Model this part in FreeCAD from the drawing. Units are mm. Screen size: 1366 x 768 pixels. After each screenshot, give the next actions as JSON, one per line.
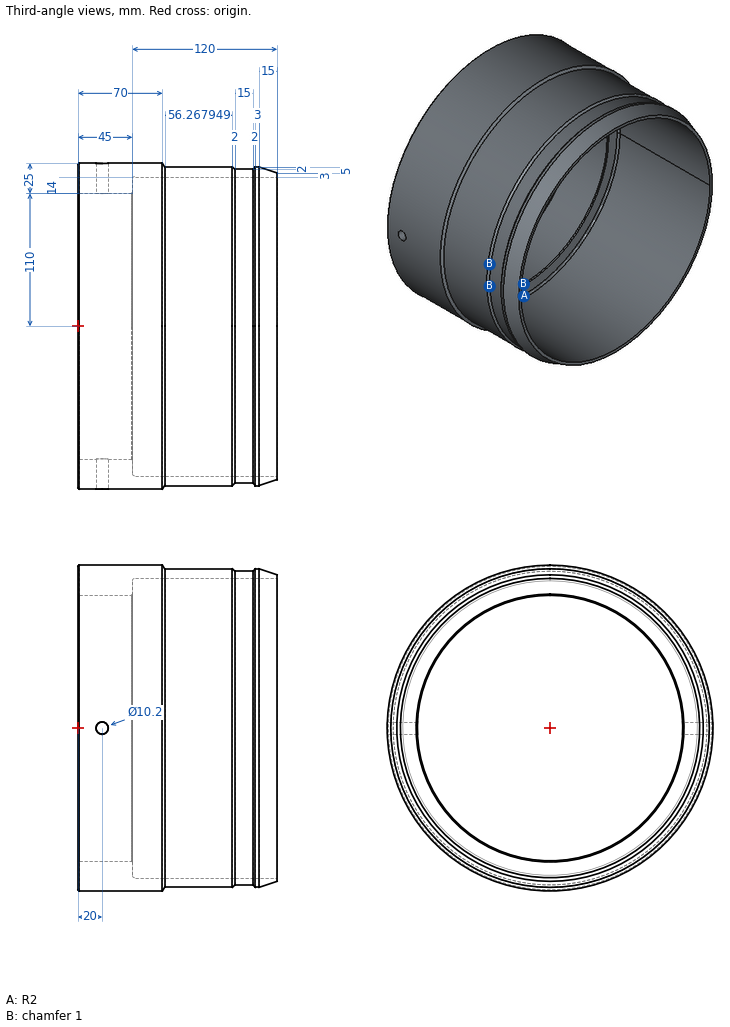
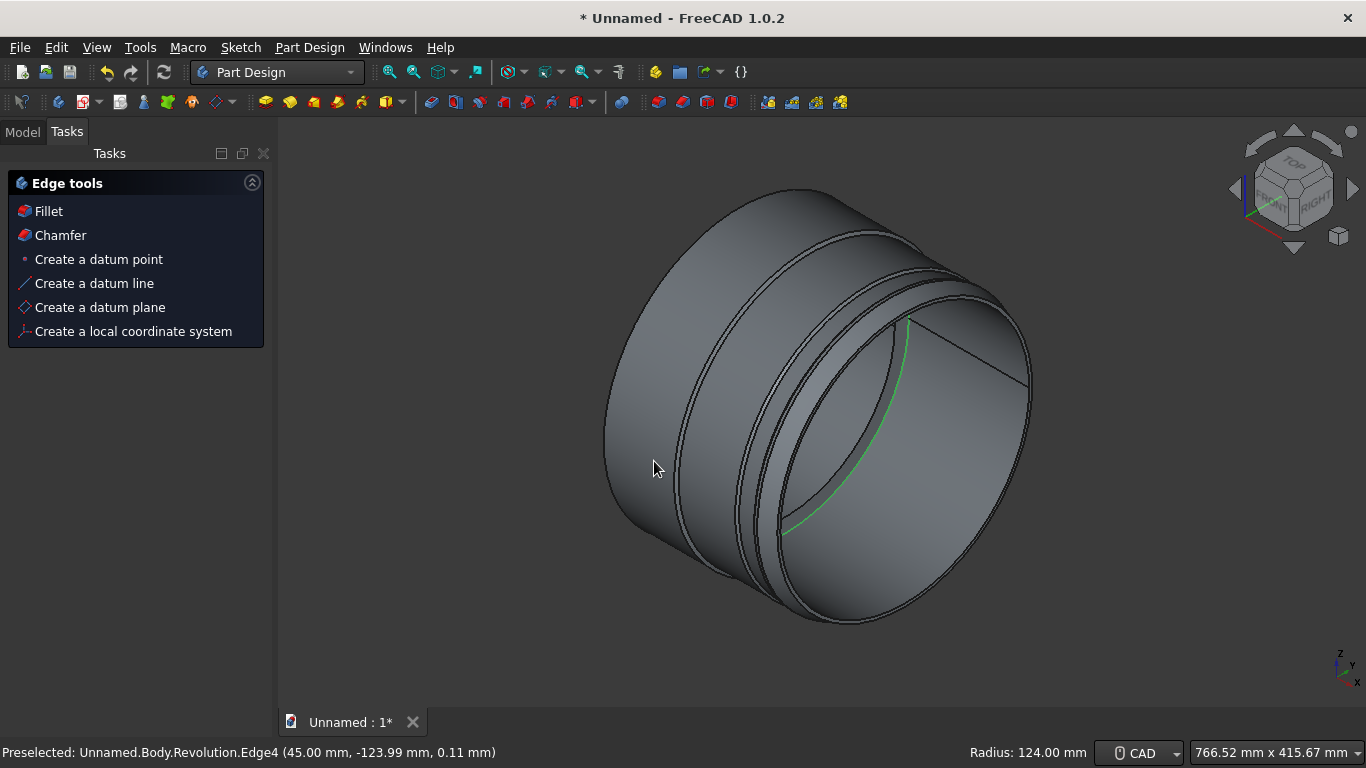
{"action": "left_click", "coordinate": [660, 102]}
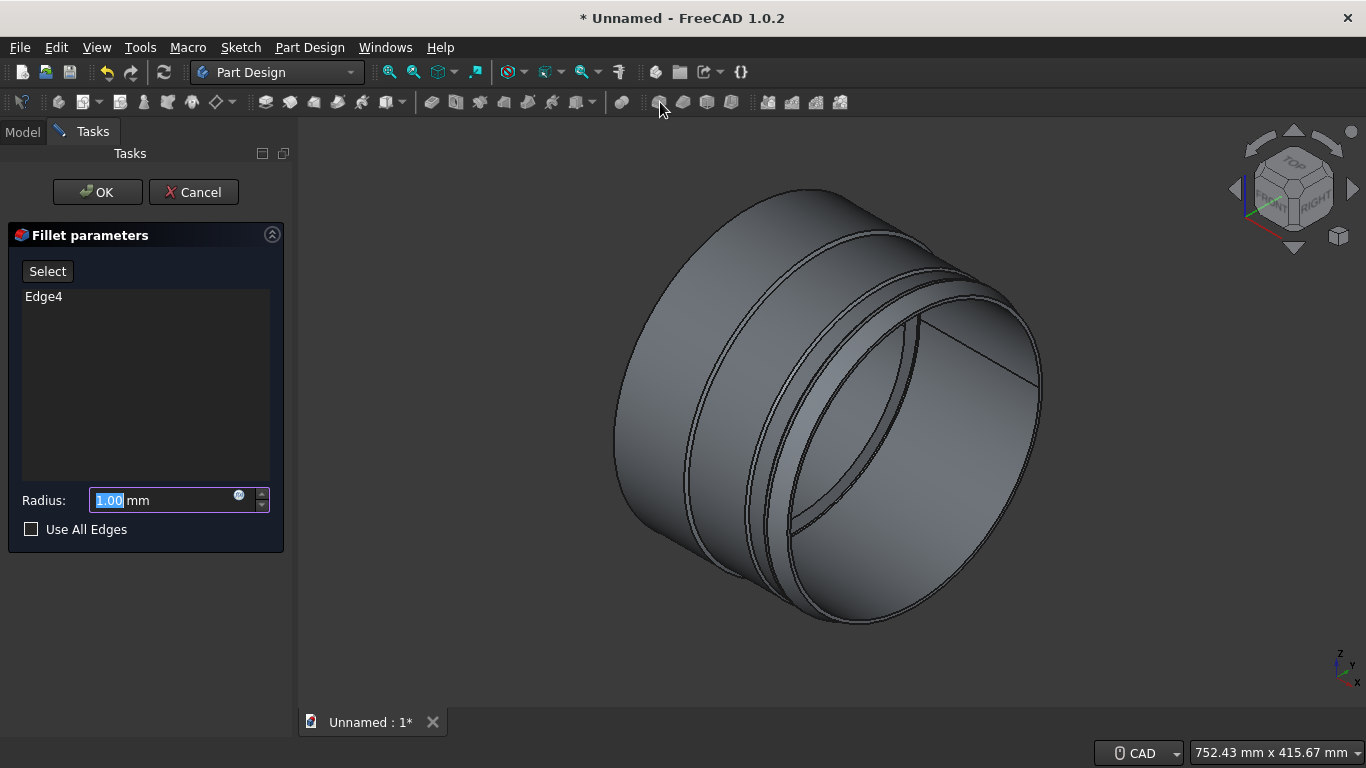
{"action": "type", "text": "2"}
{"action": "key", "text": "Tab"}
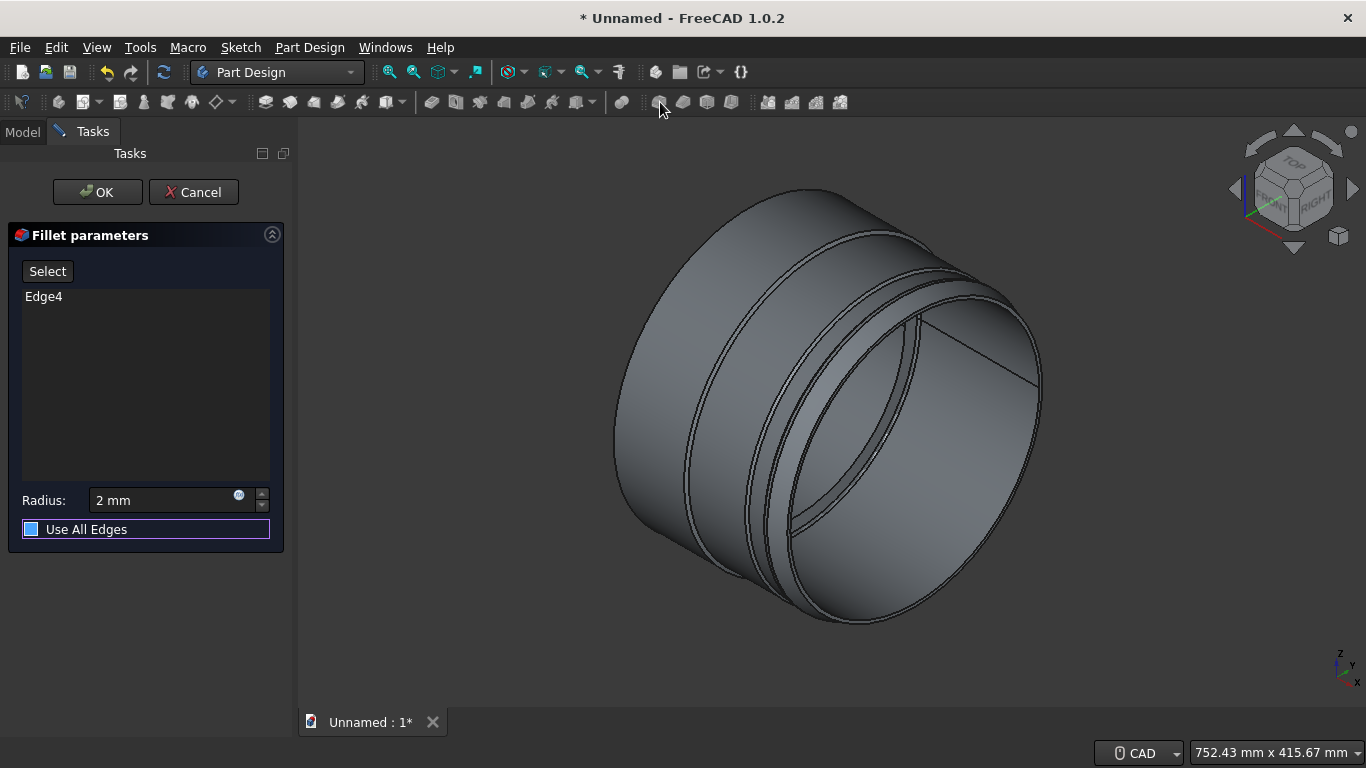
{"action": "left_click", "coordinate": [98, 192]}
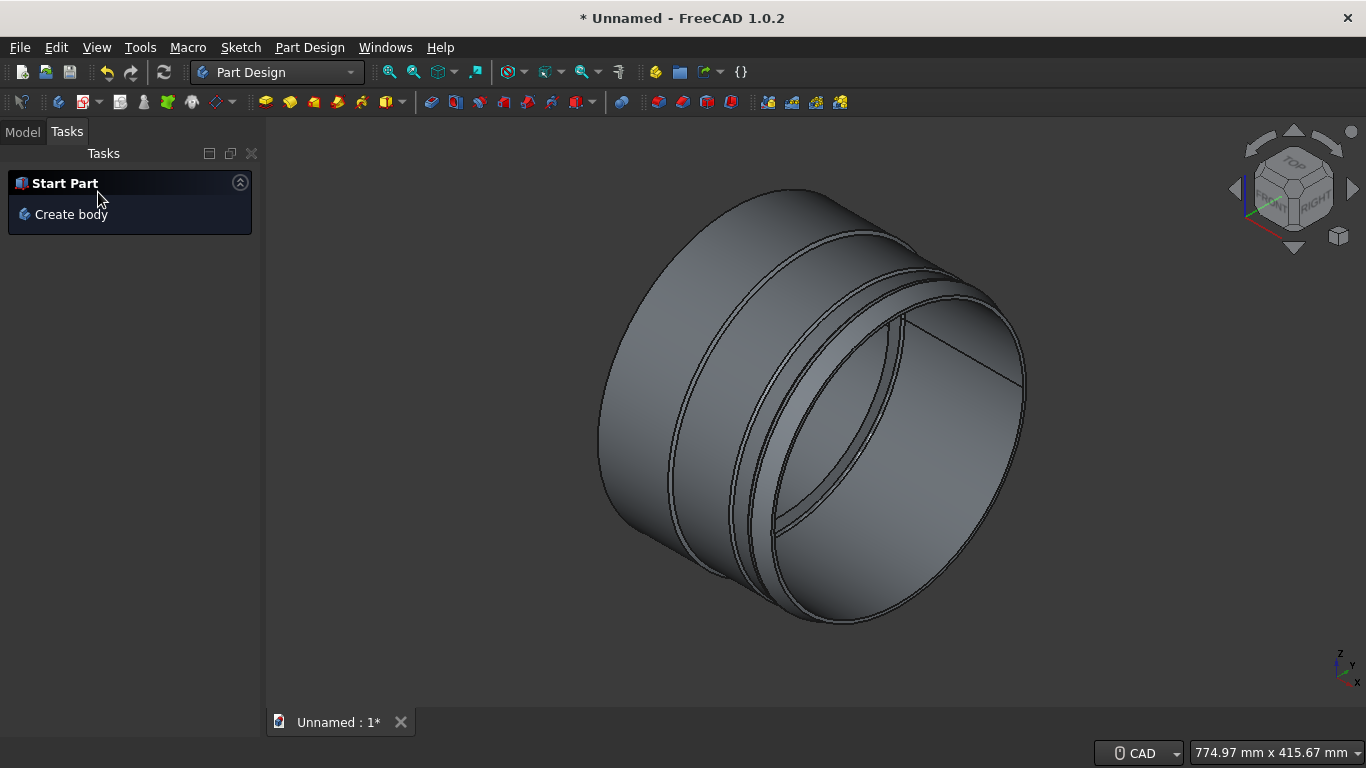
{"action": "left_click", "coordinate": [812, 491]}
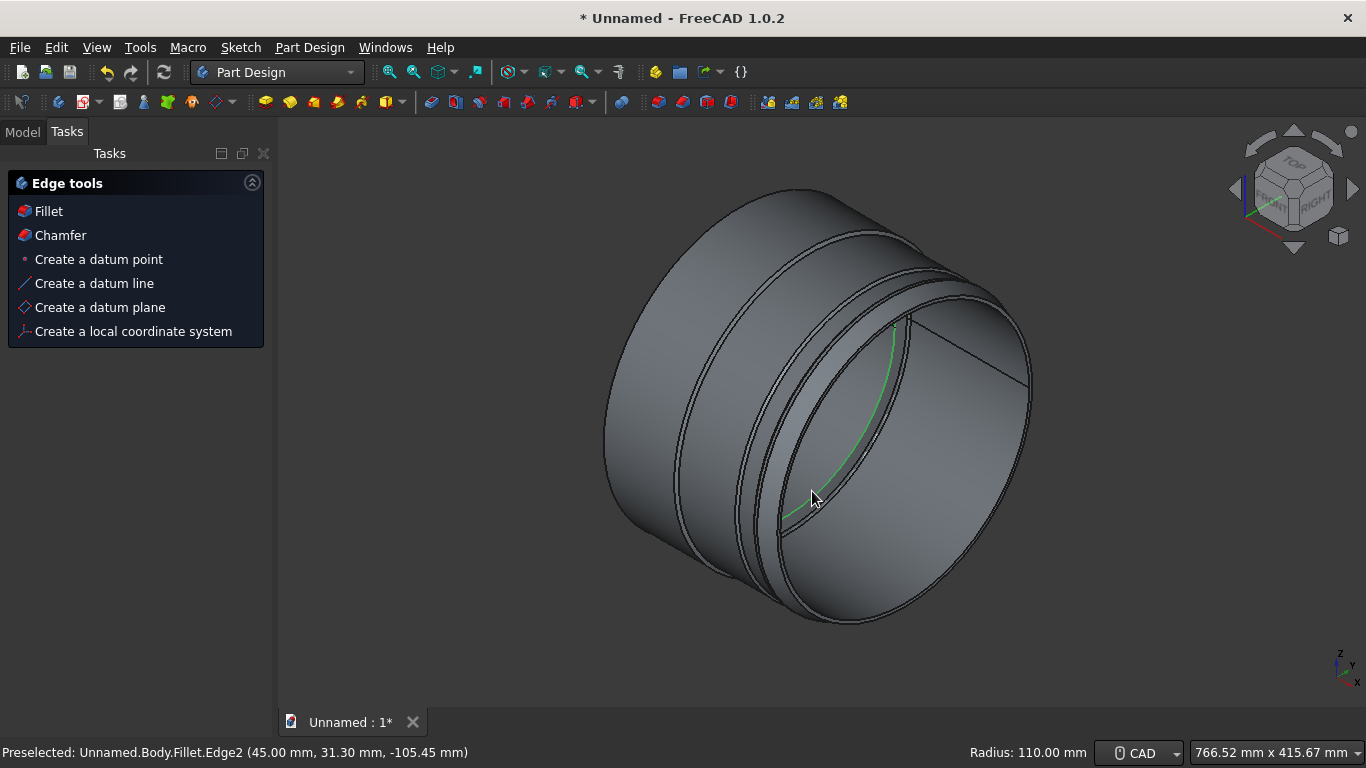
{"action": "key", "text": "2"}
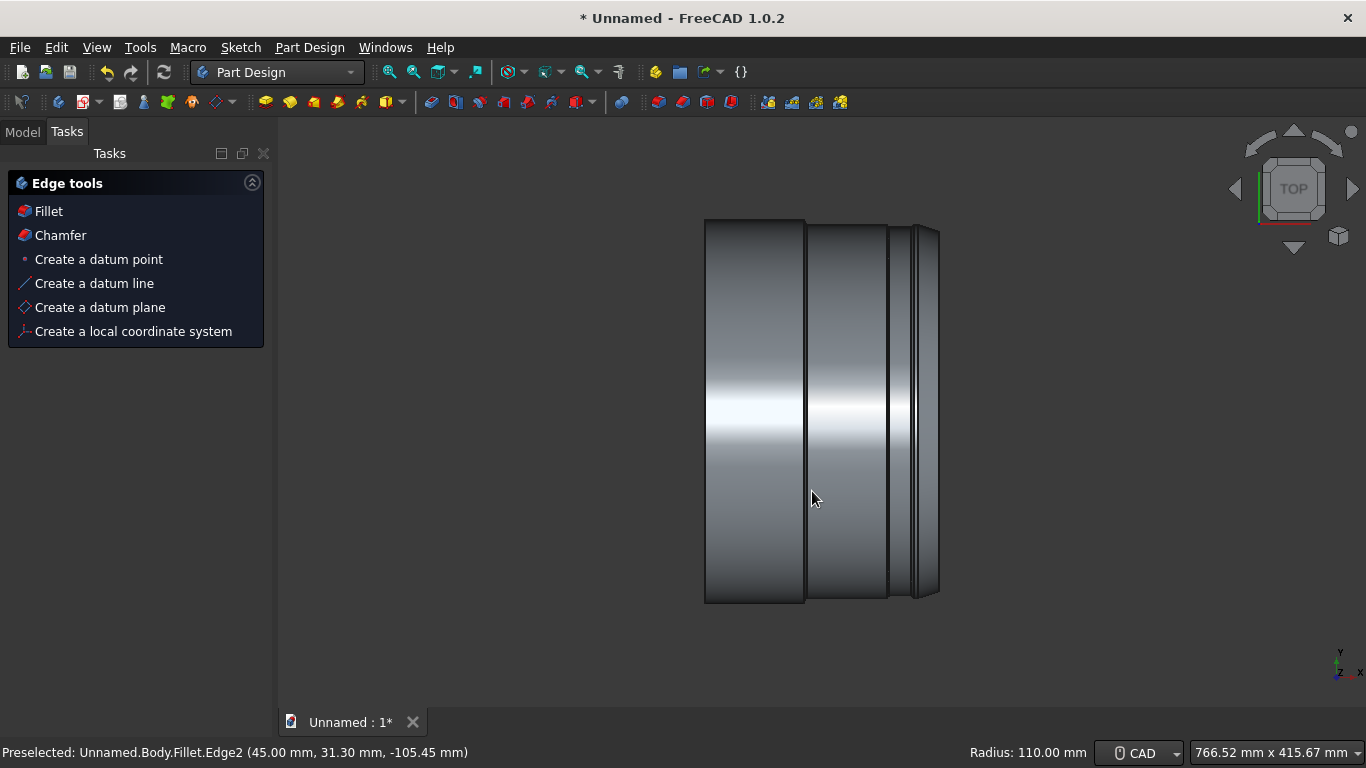
{"action": "left_click", "coordinate": [705, 566], "text": "ctrl"}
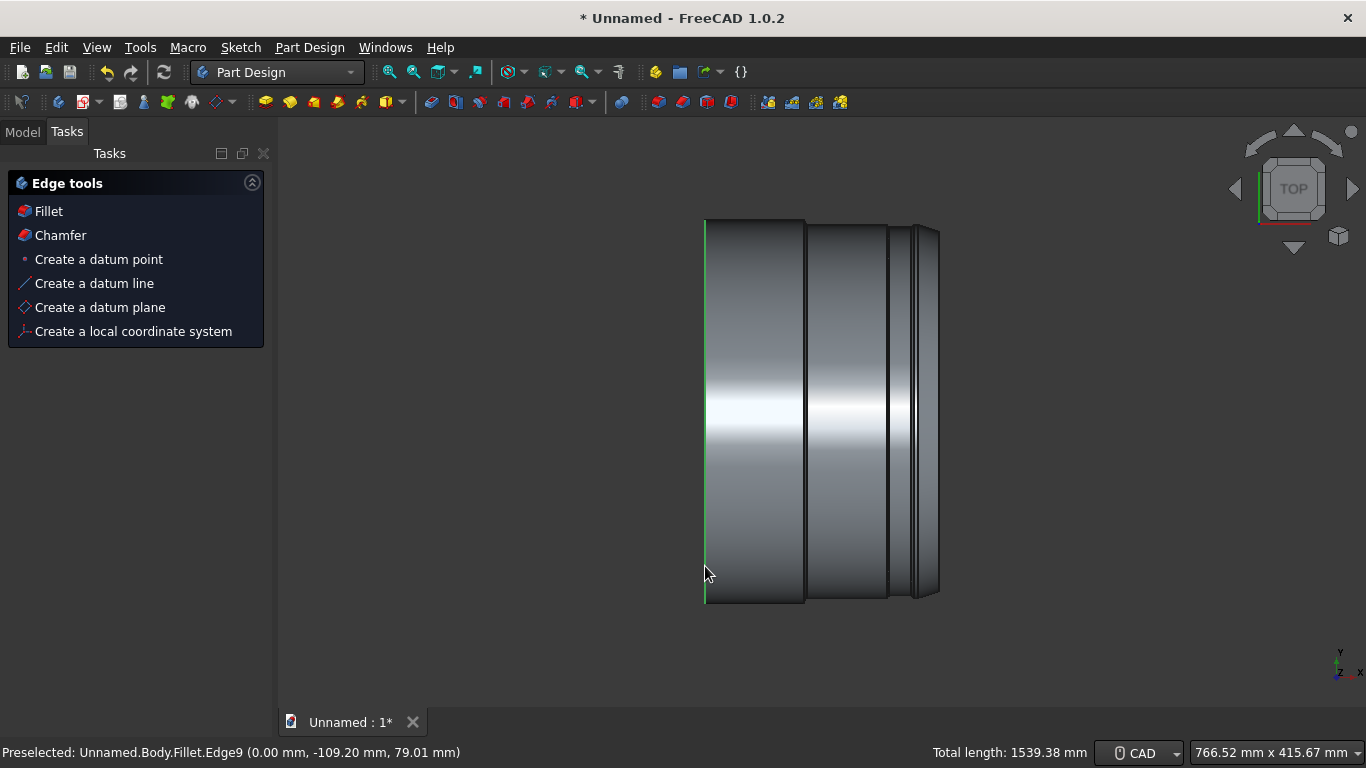
{"action": "key", "text": "0"}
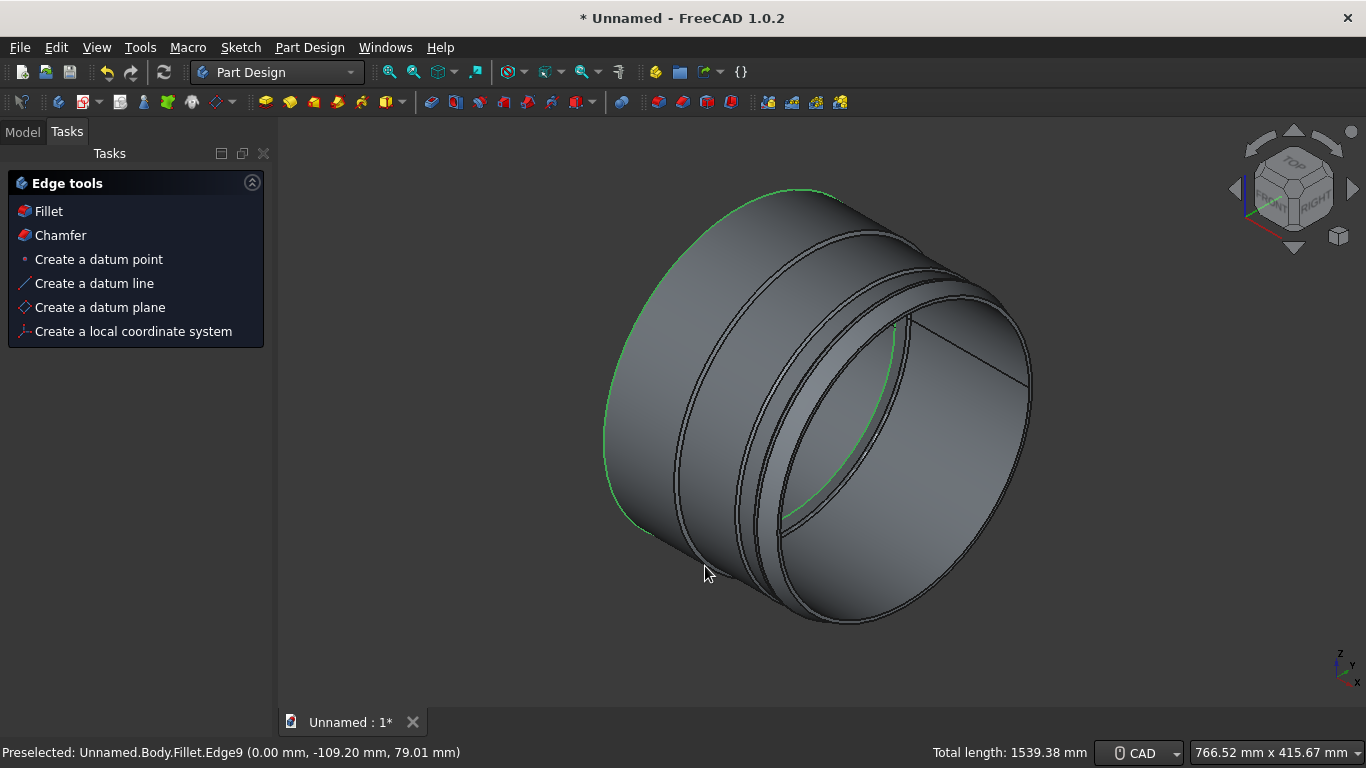
{"action": "key", "text": "1"}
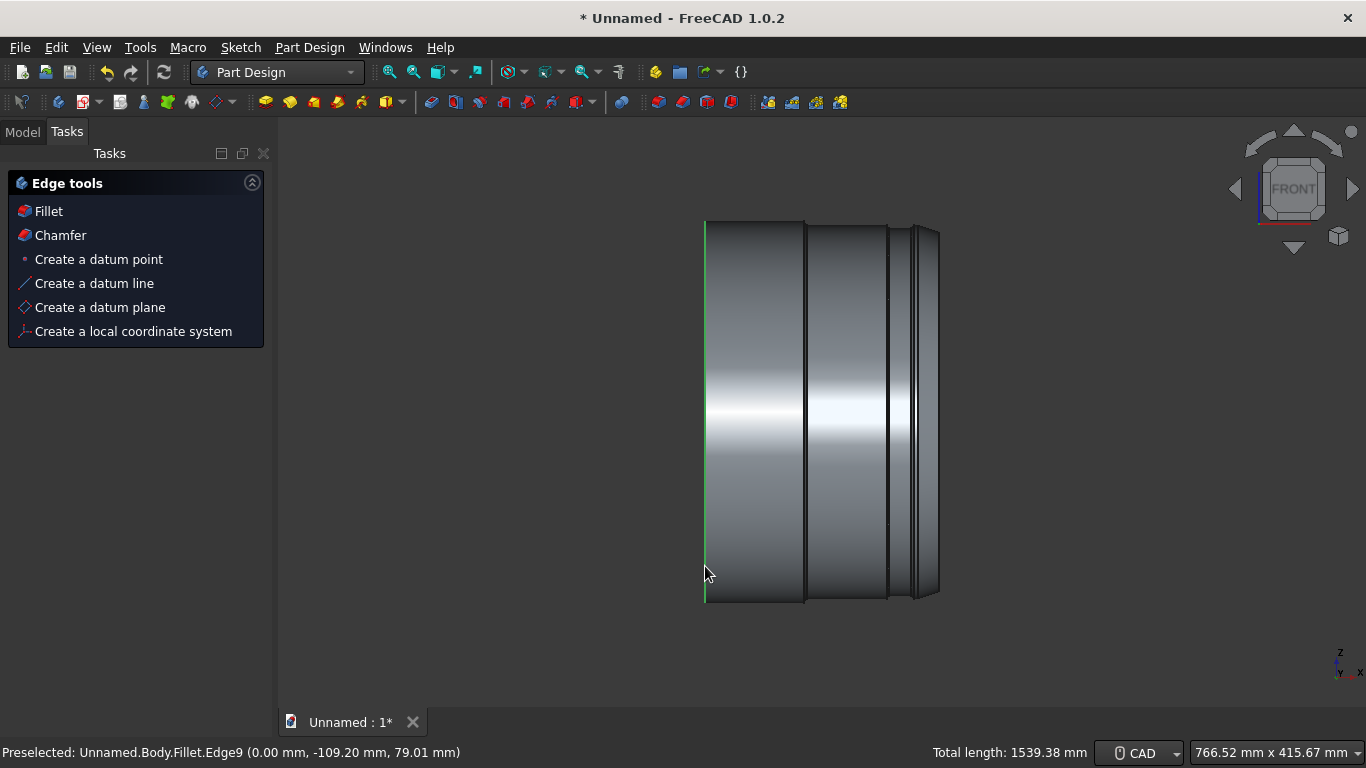
{"action": "key", "text": "3"}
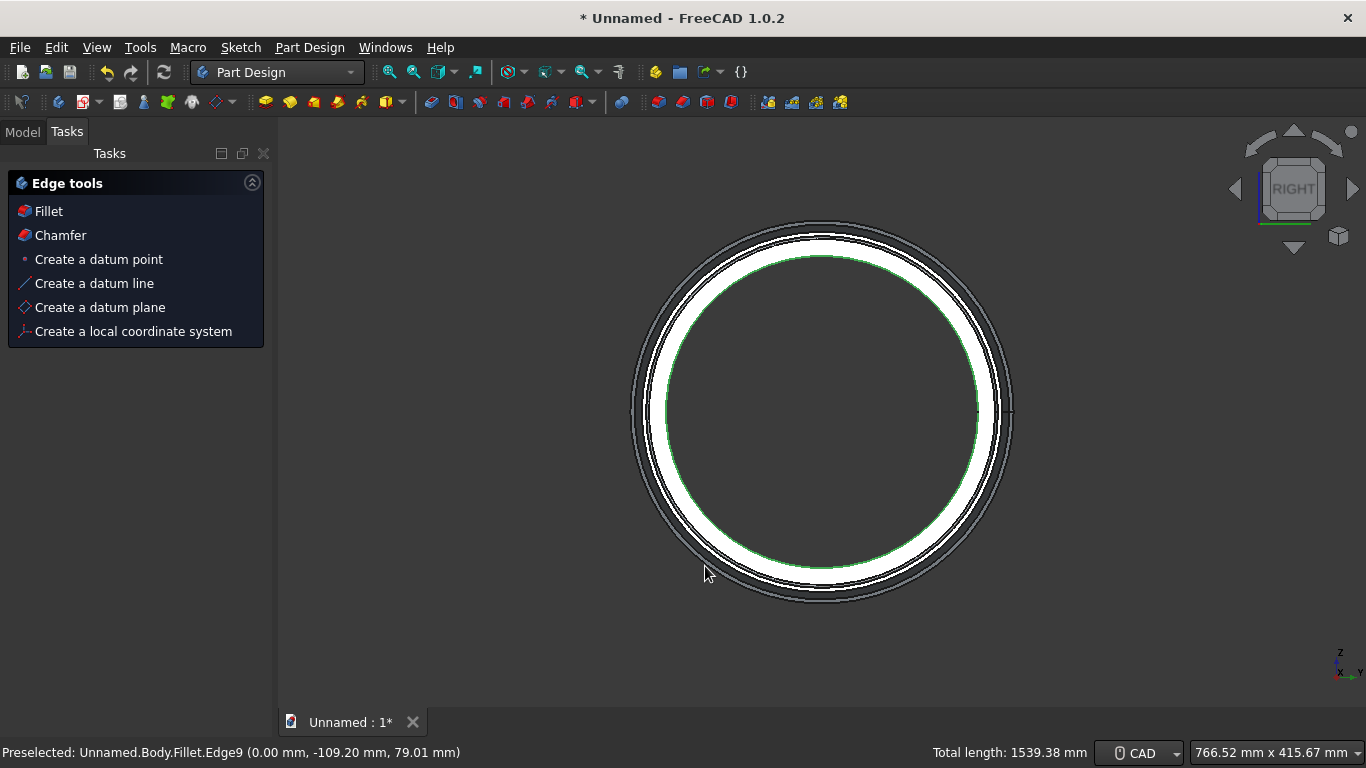
{"action": "key", "text": "5"}